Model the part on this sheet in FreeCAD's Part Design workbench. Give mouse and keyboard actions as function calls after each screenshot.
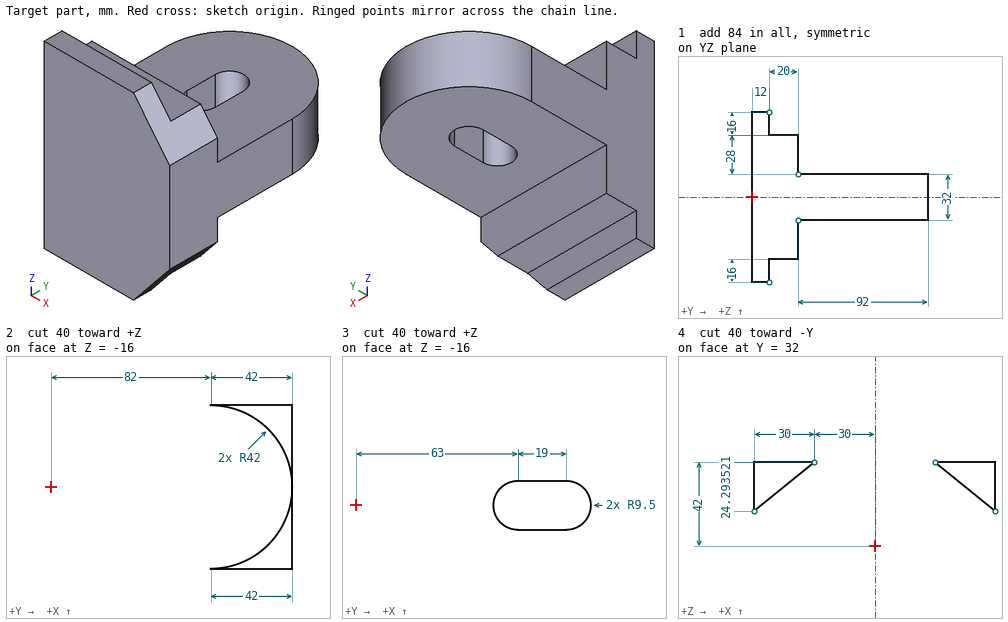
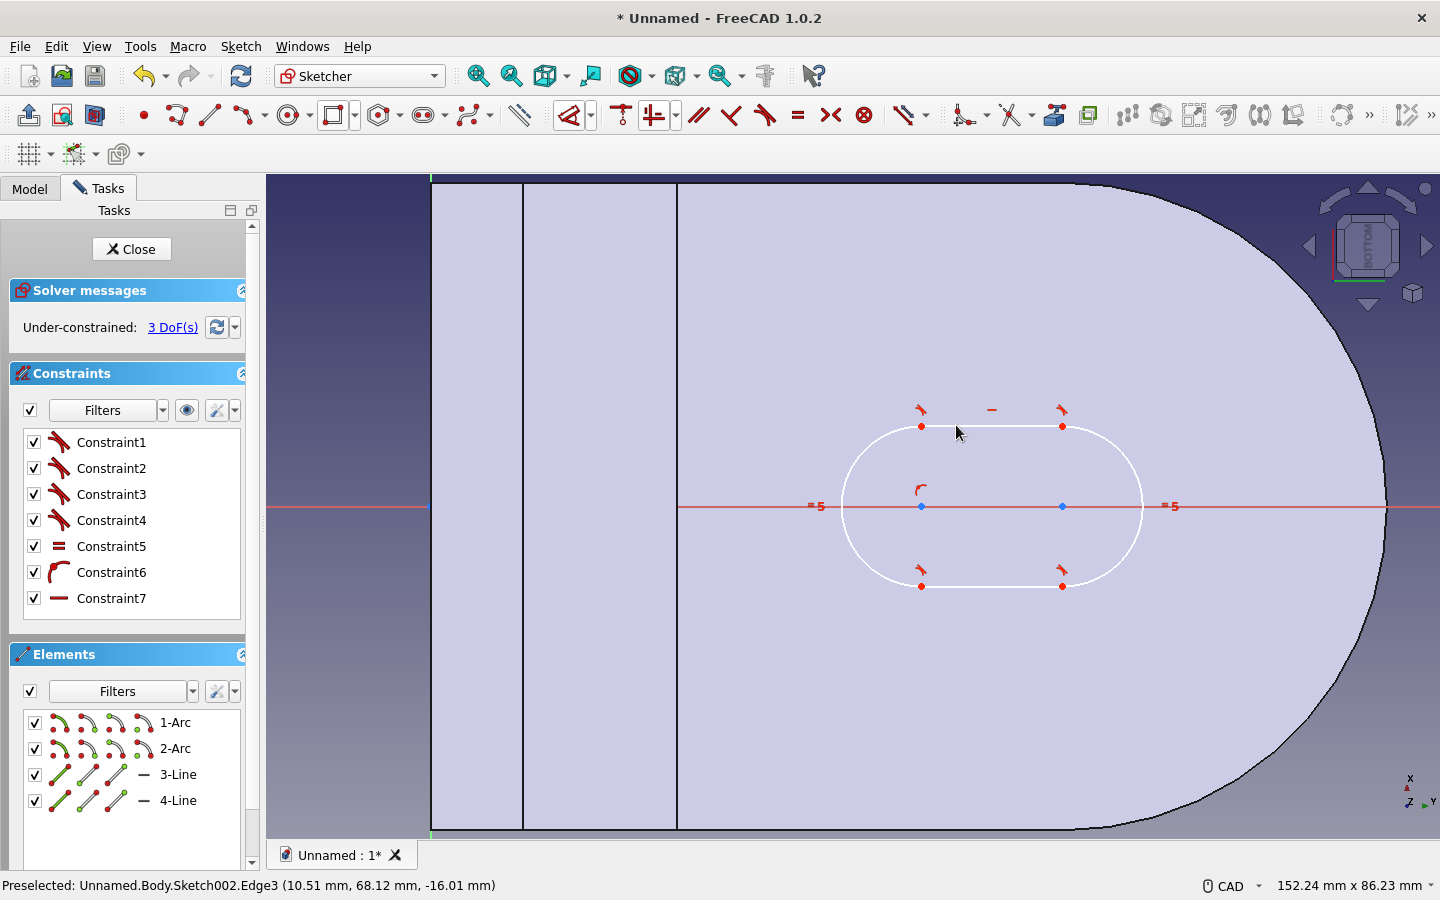
click(857, 459)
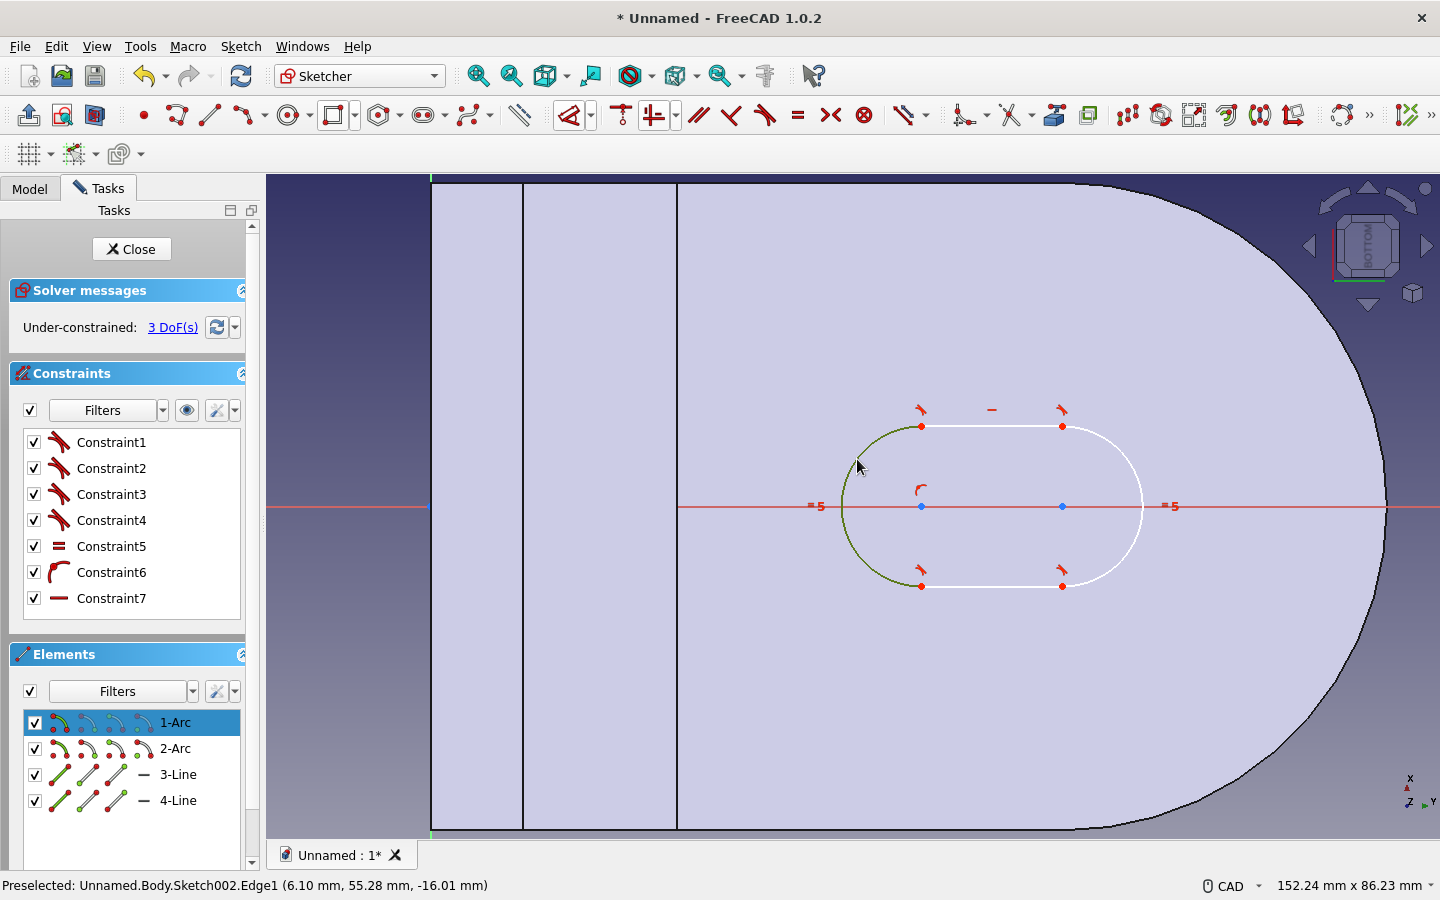
key(k)
key(r)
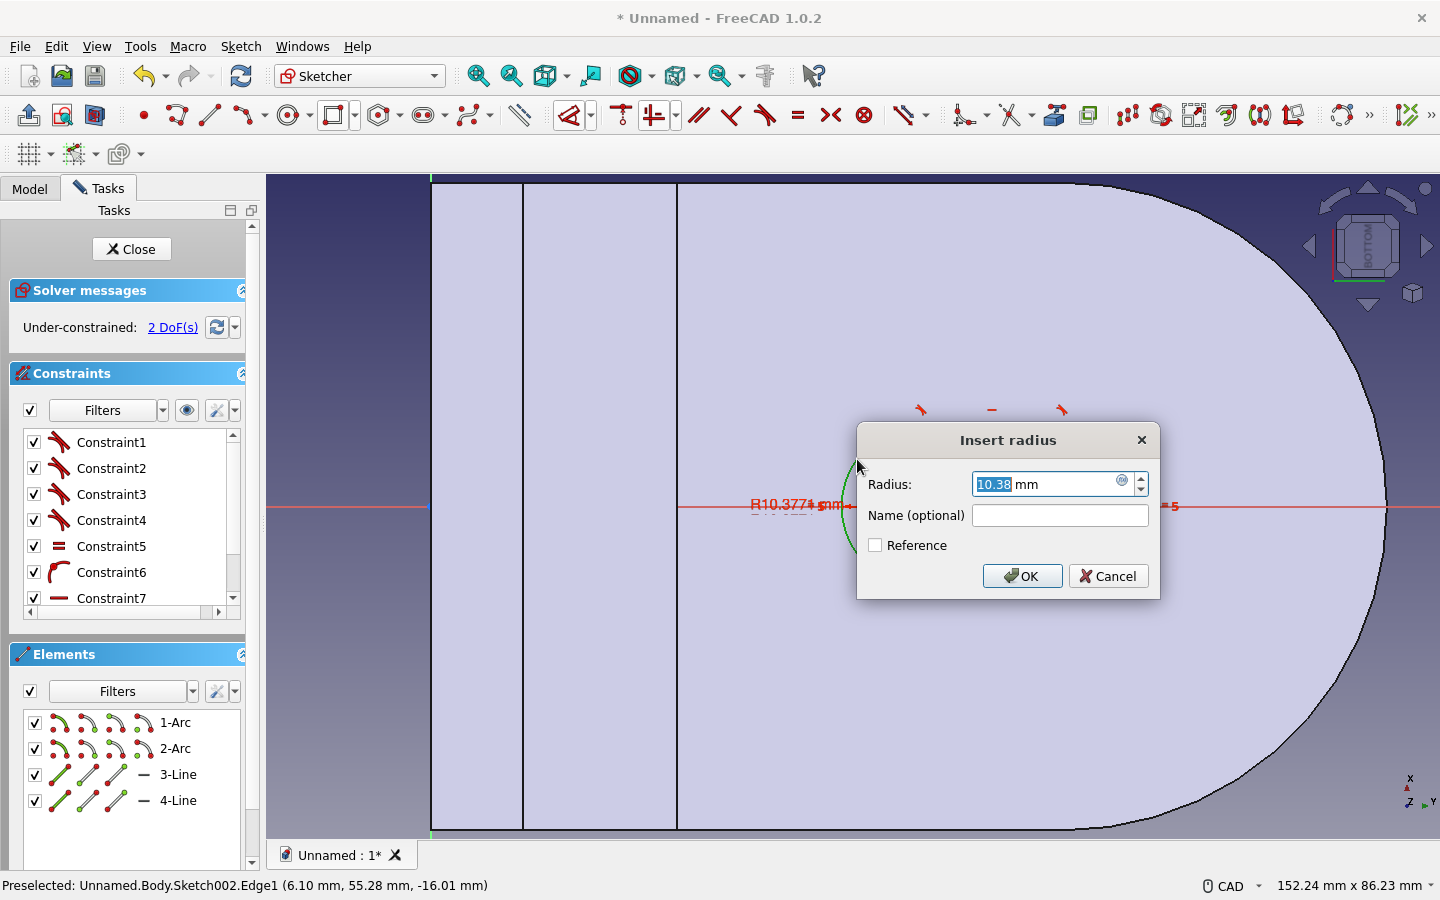
text(9.5)
key(Return)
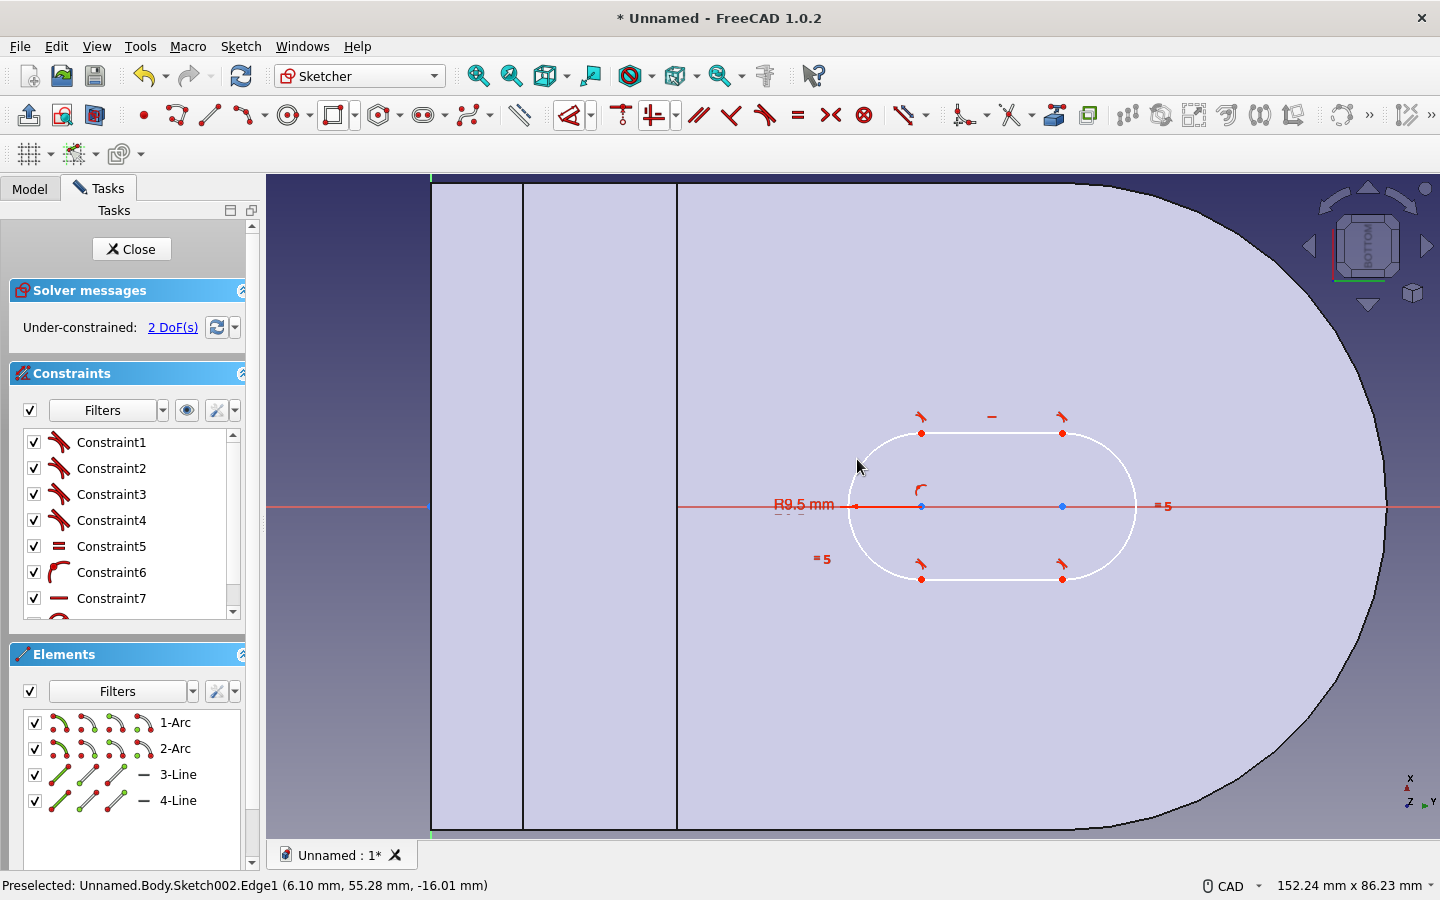
click(964, 433)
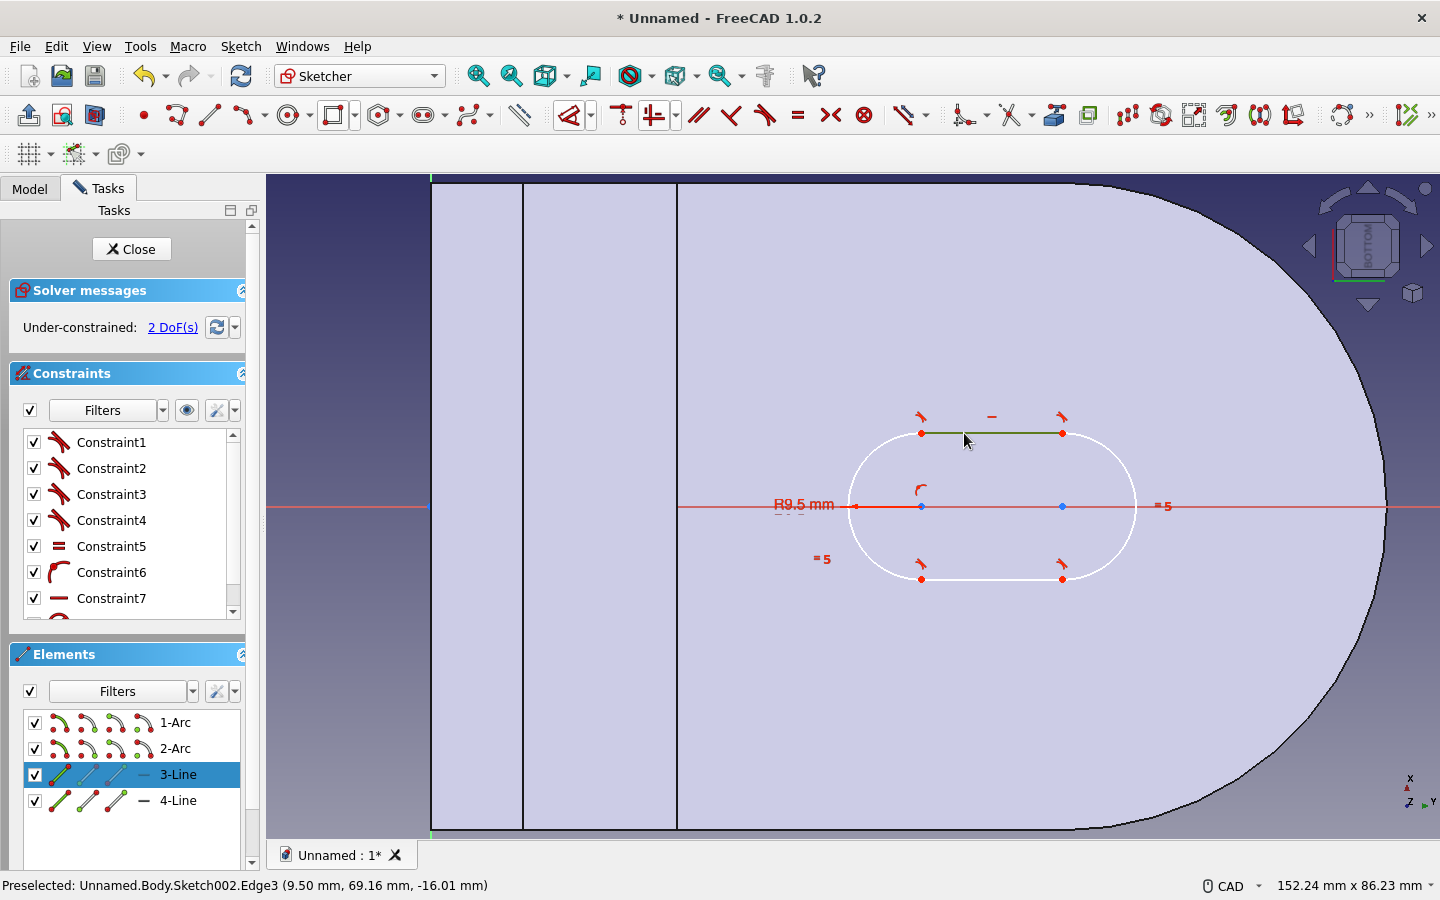
key(l)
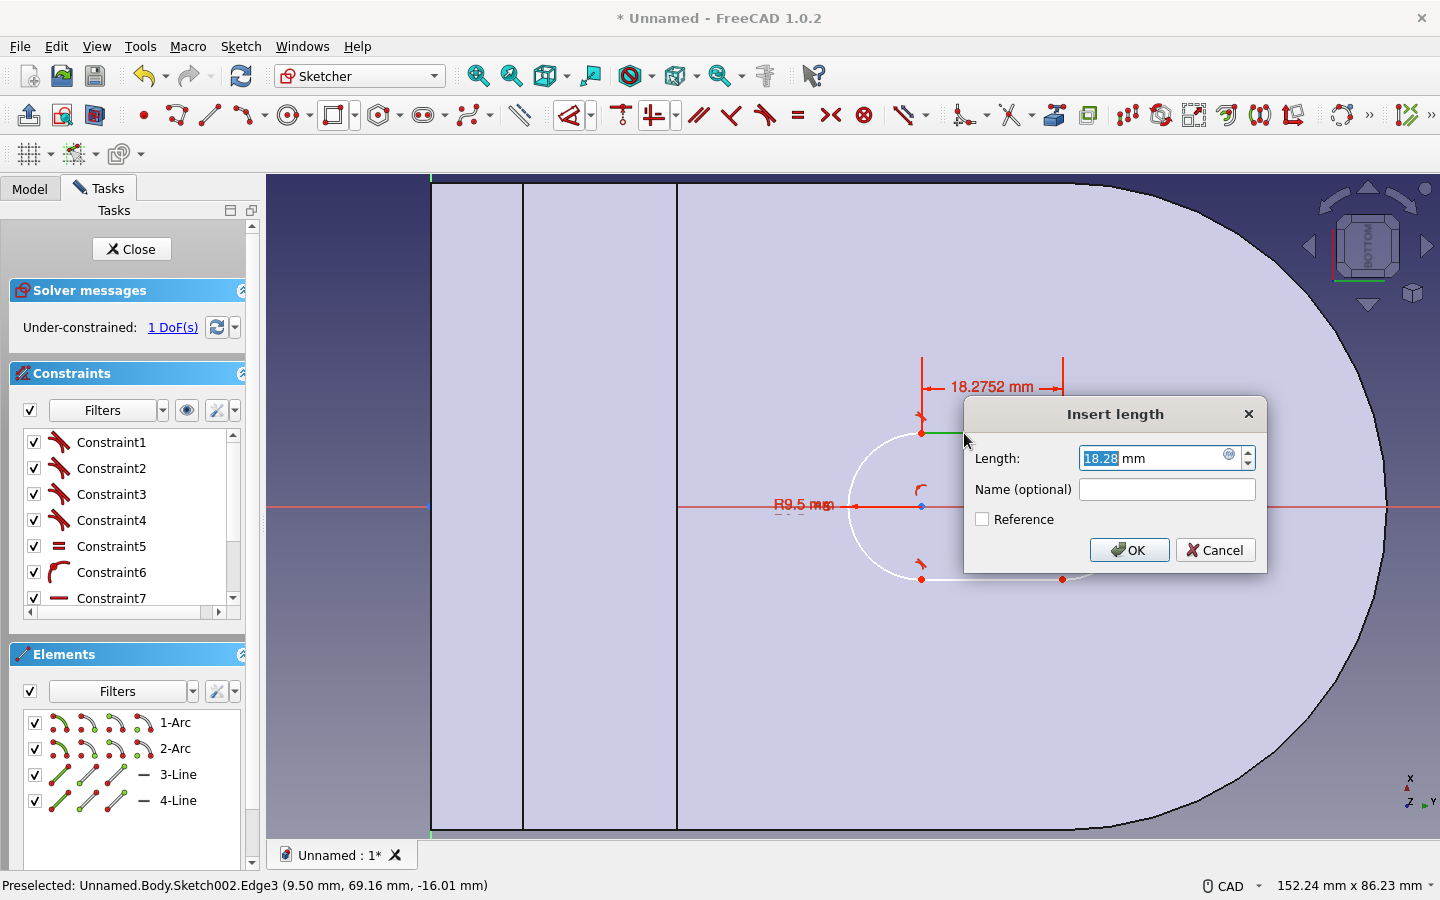
text(19)
key(Return)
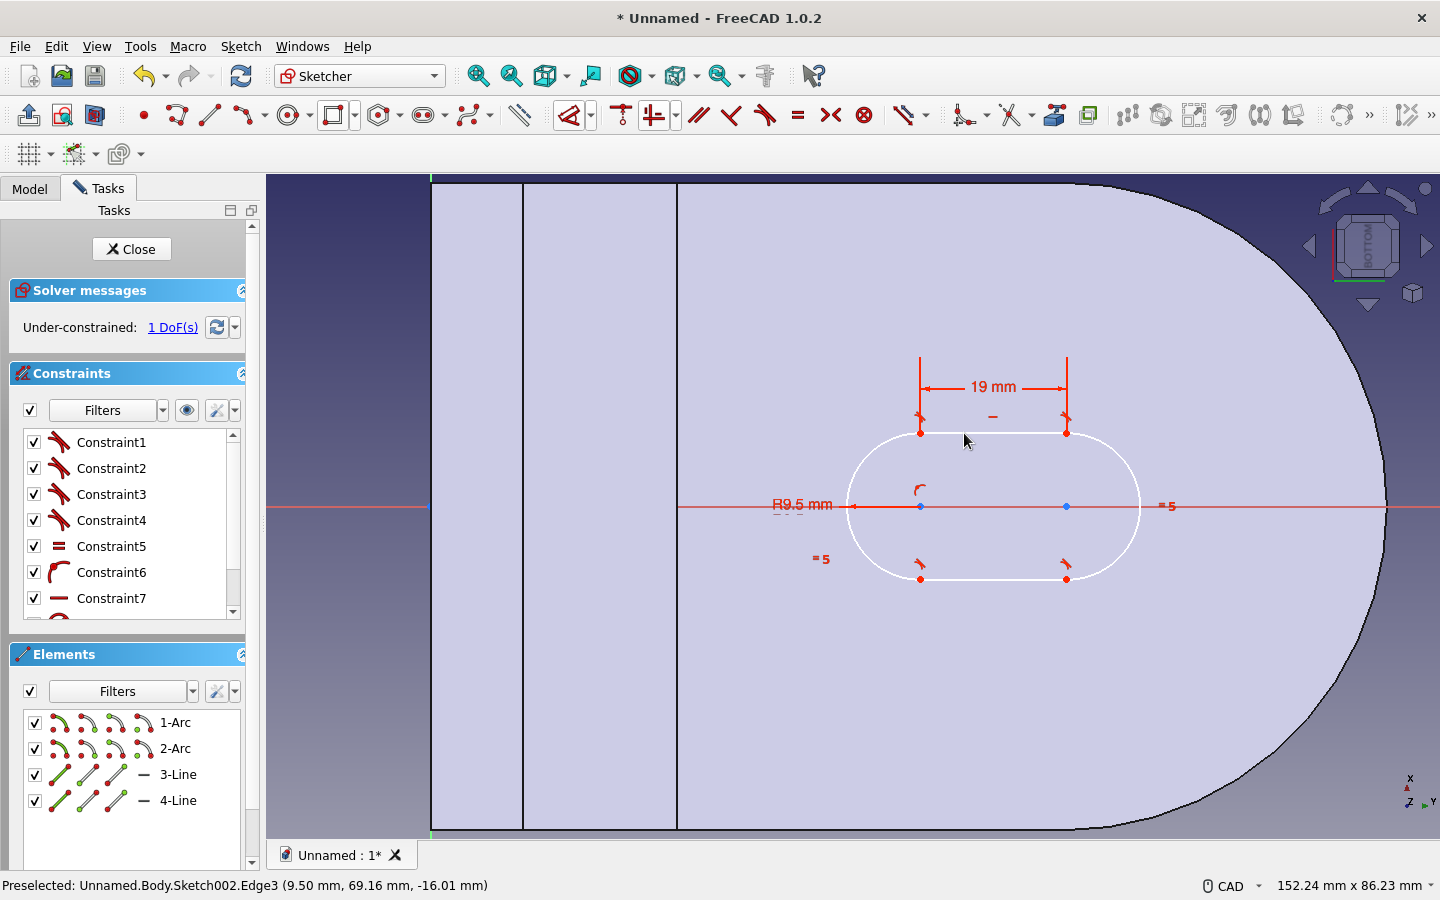
click(920, 433)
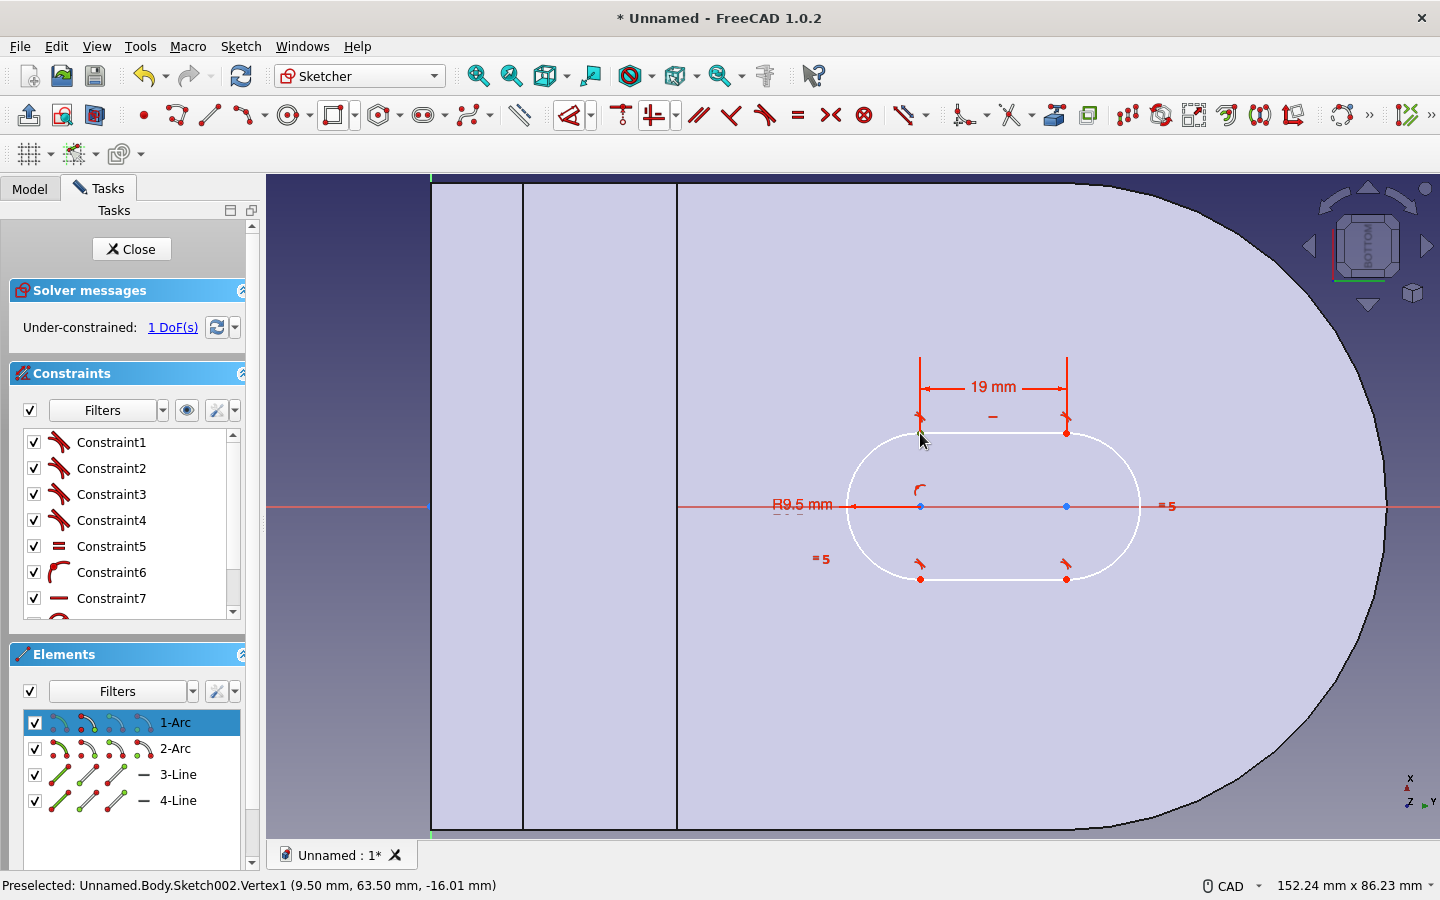
click(590, 116)